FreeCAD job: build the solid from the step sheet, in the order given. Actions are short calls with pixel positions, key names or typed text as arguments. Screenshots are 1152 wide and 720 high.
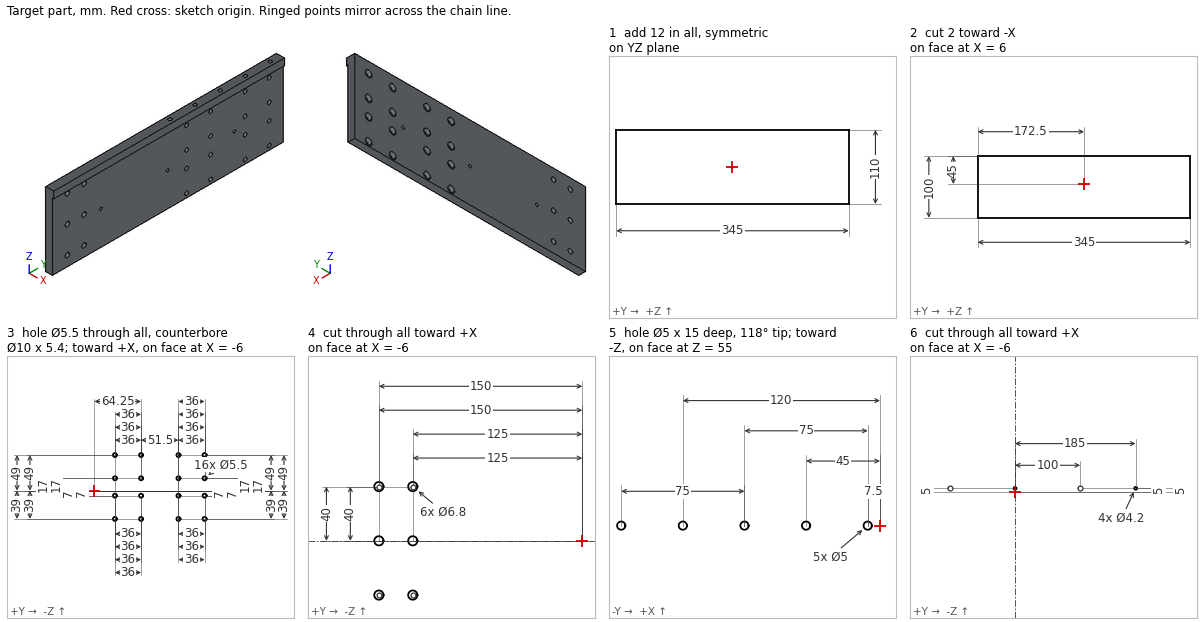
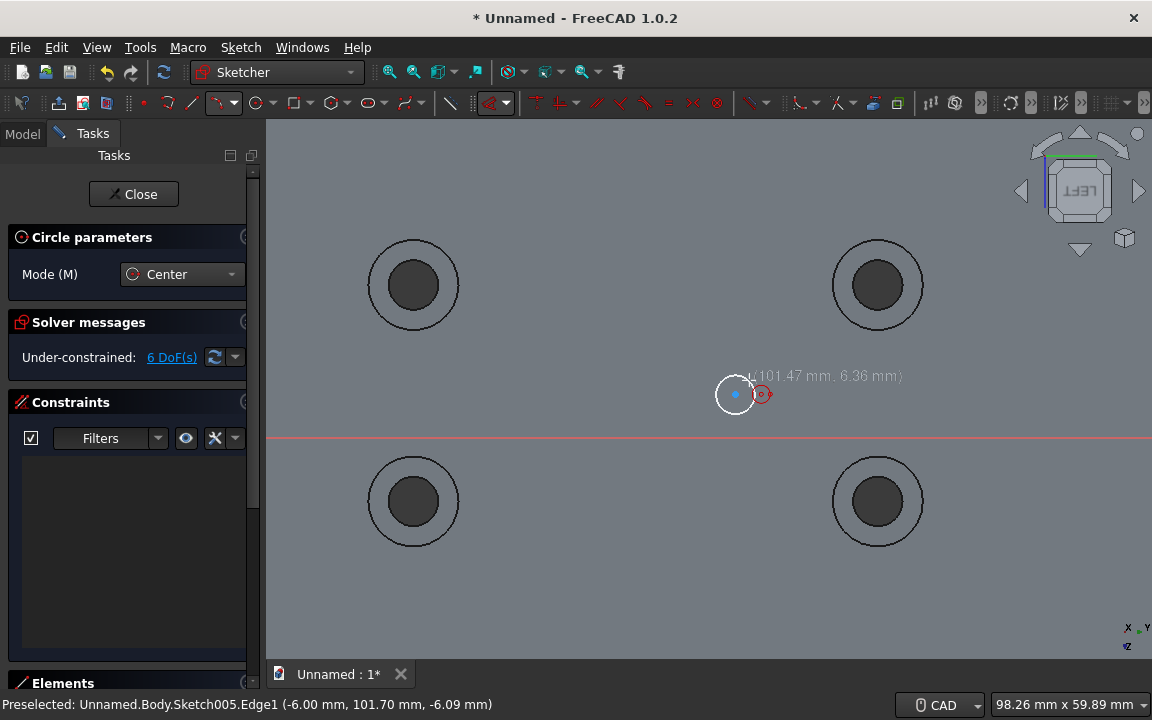
scroll(748, 385, down, 8)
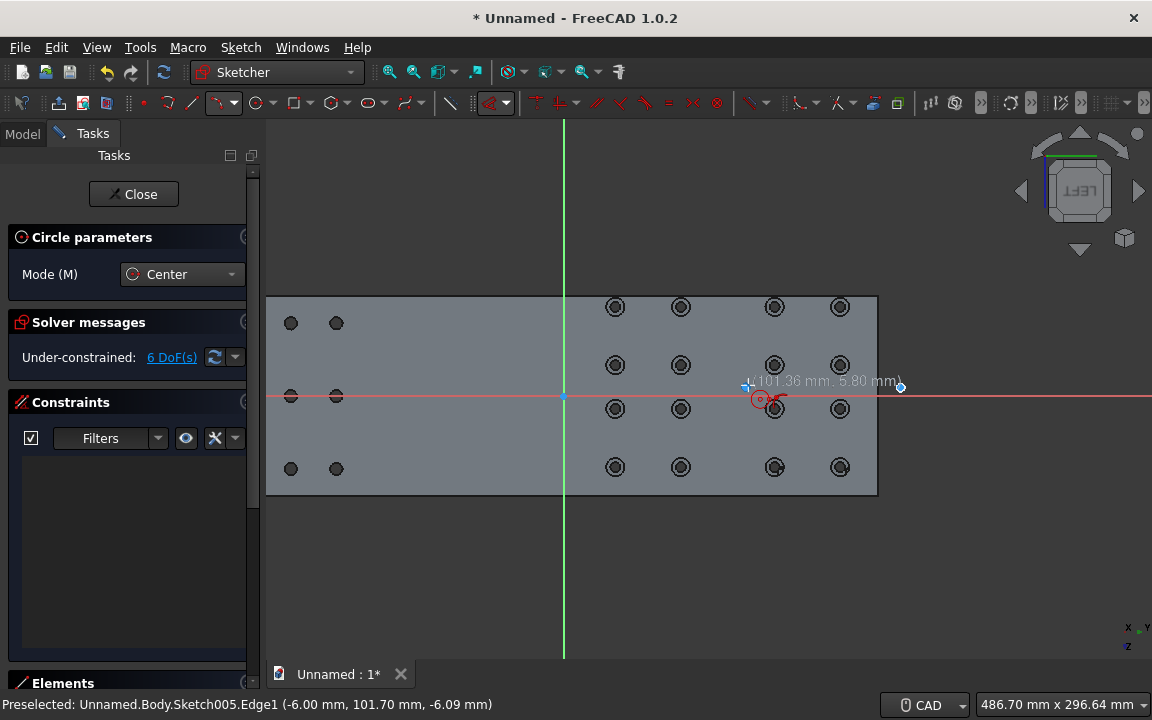
scroll(564, 387, up, 9)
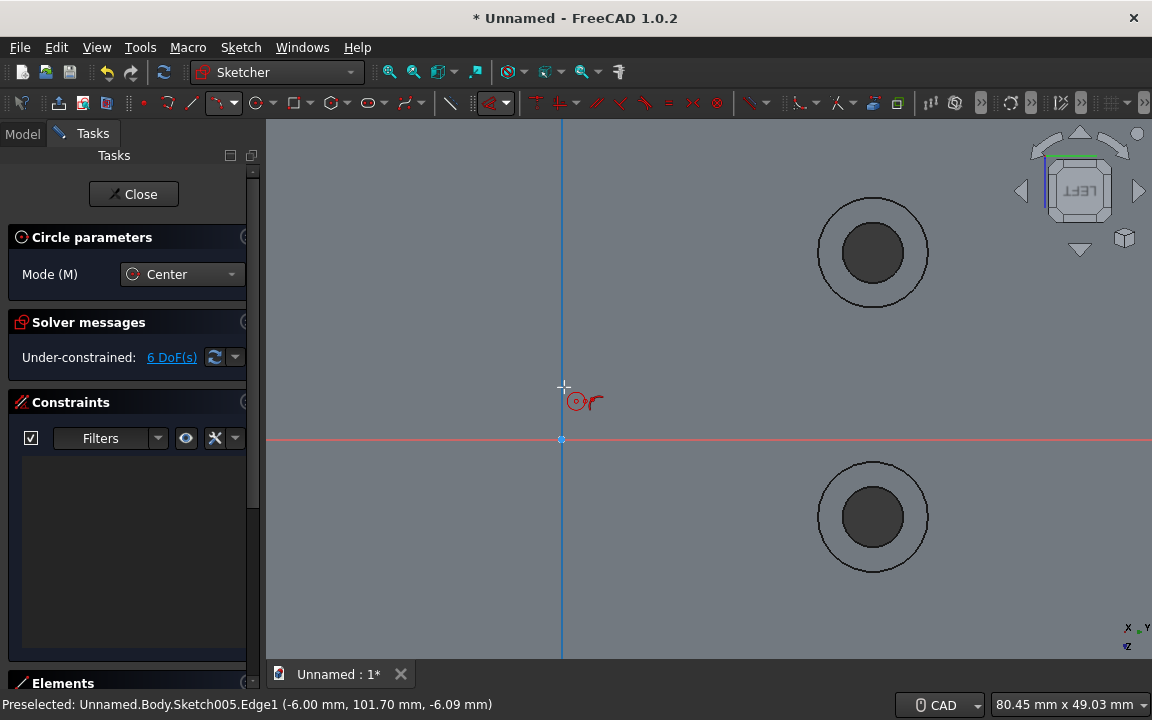
scroll(563, 387, down, 9)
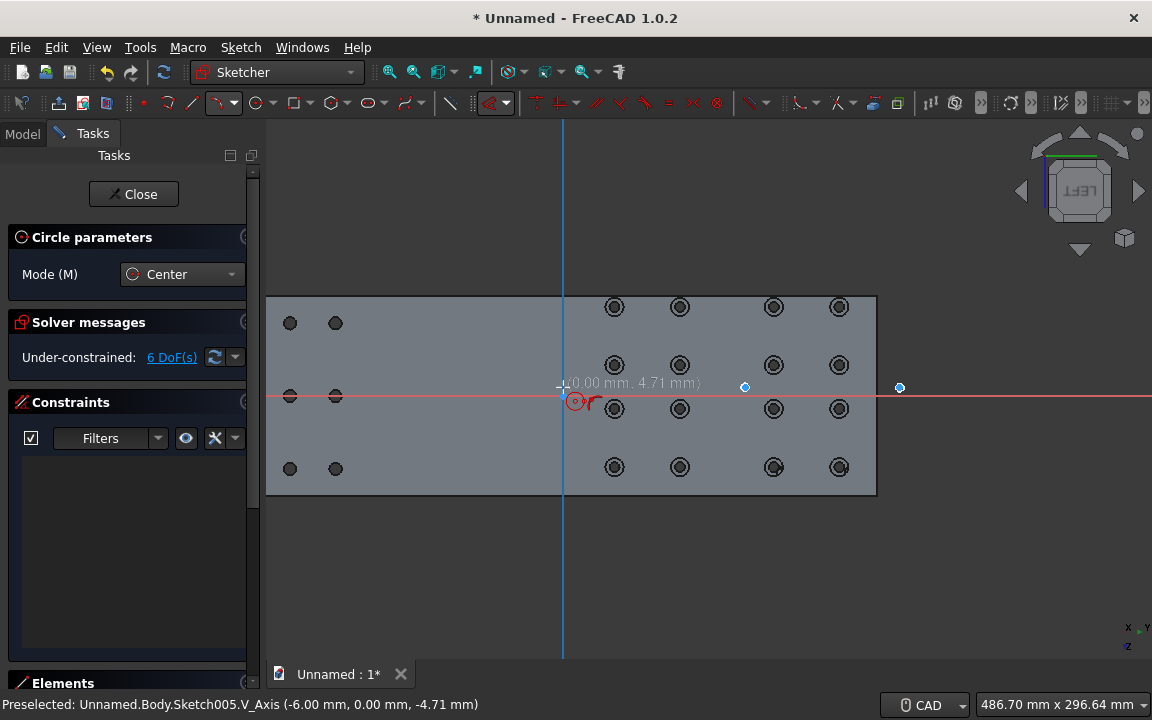
scroll(563, 387, up, 3)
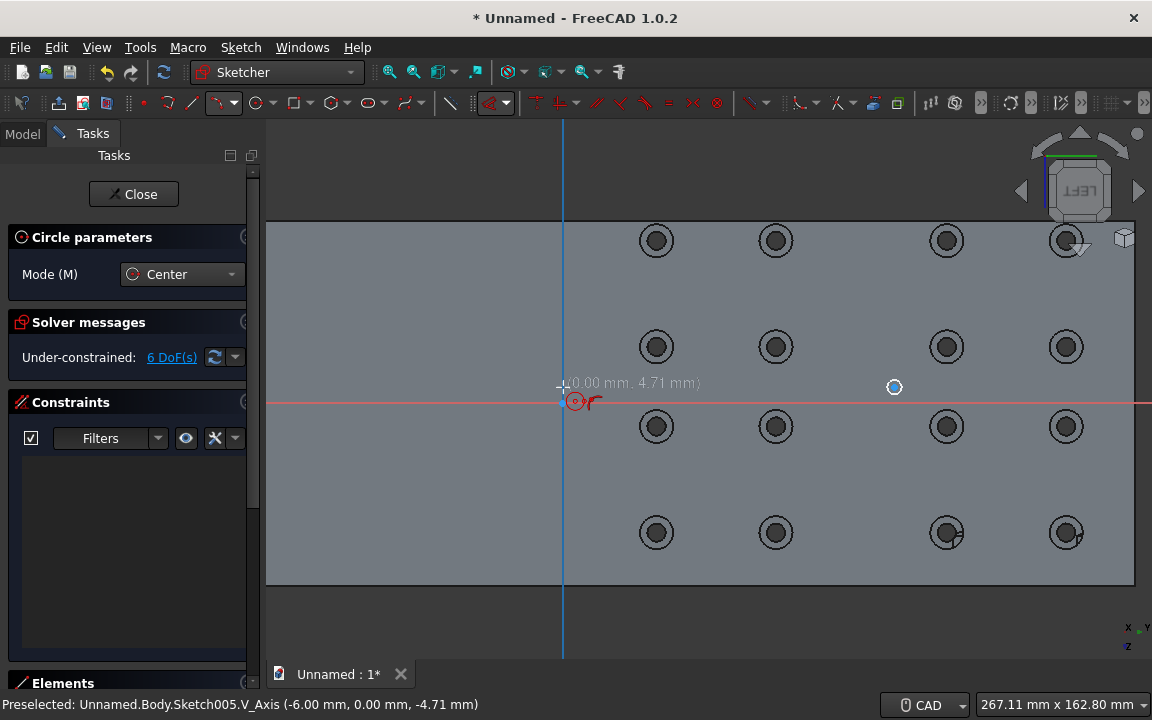
click(563, 387)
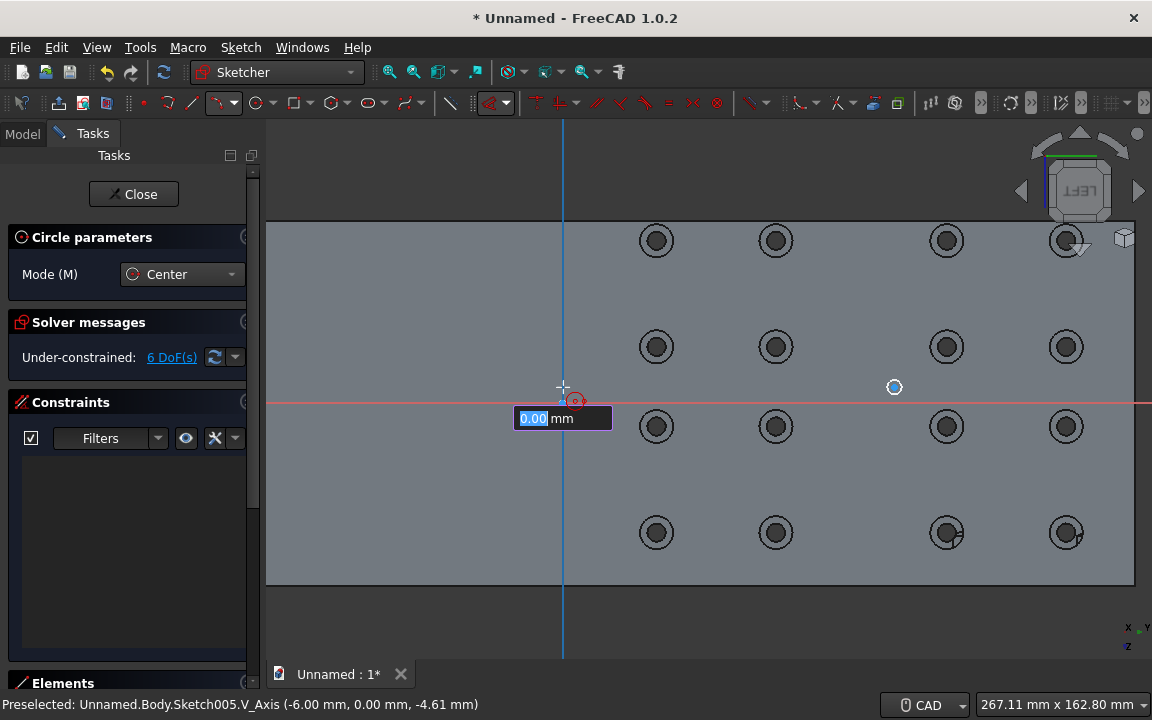
scroll(569, 384, up, 5)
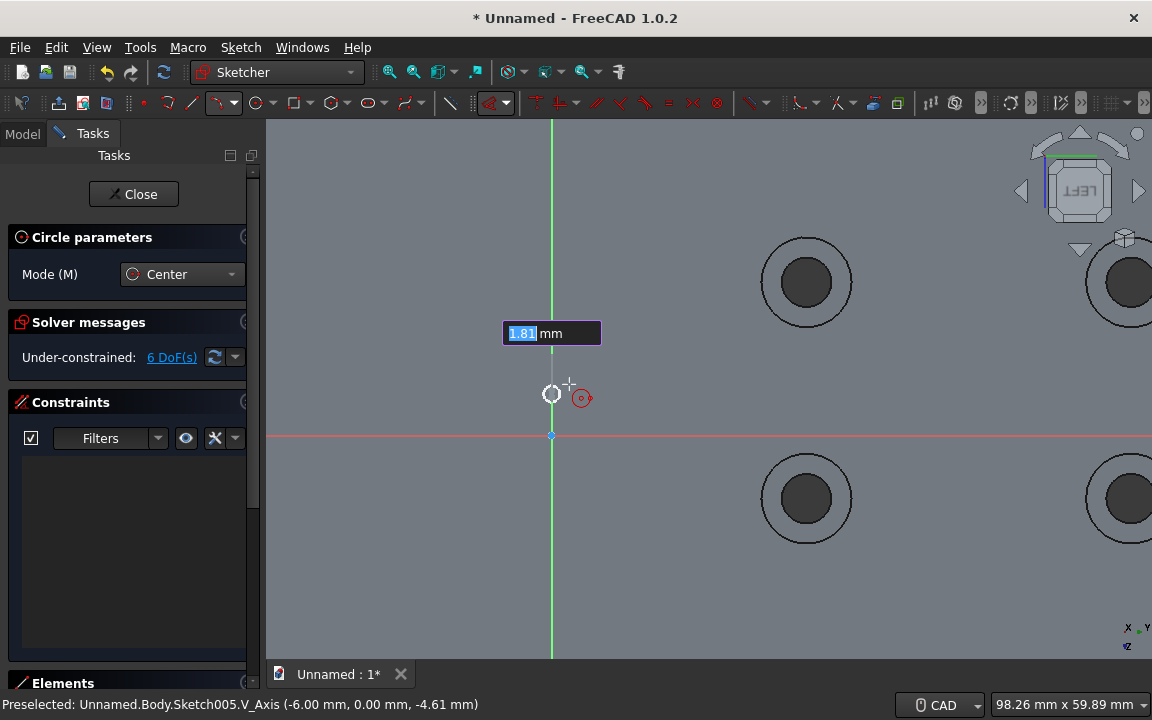
click(570, 384)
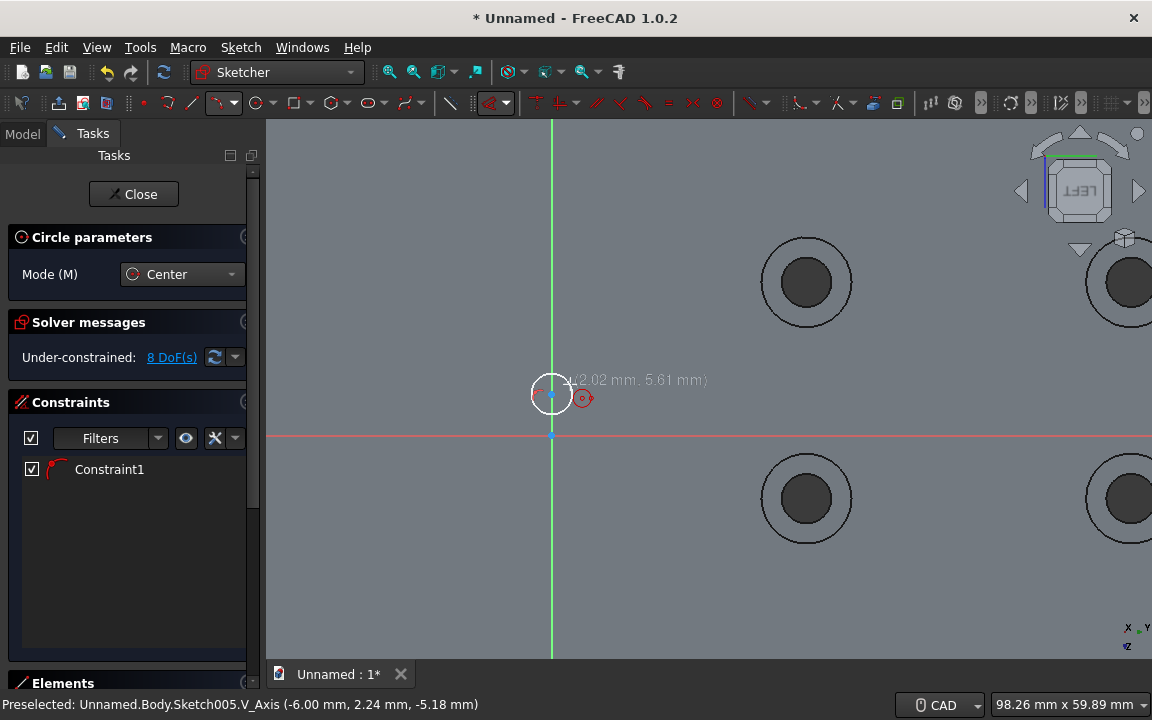
scroll(566, 385, down, 8)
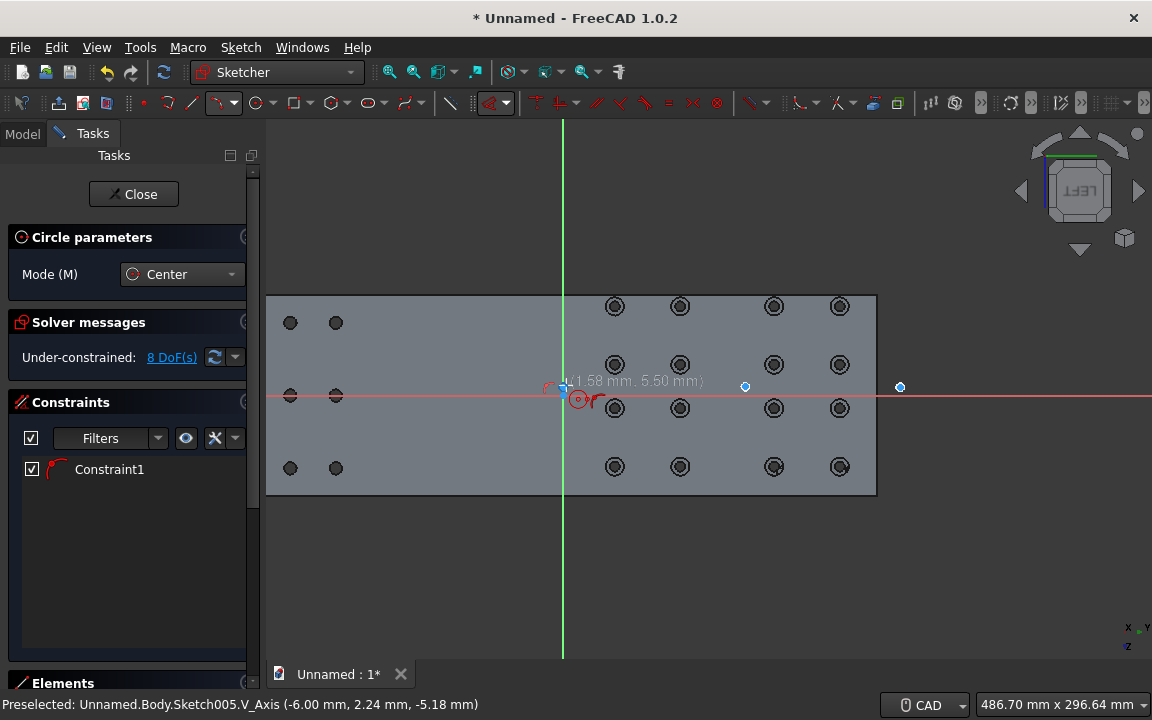
scroll(381, 386, up, 9)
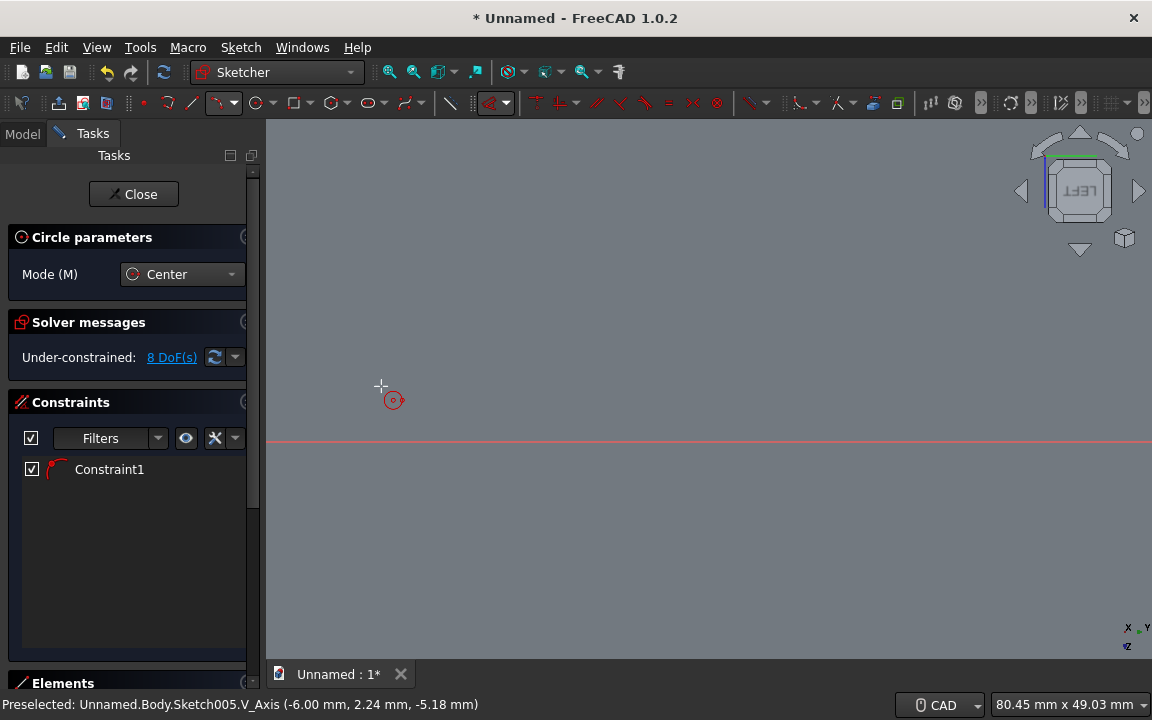
scroll(381, 386, down, 9)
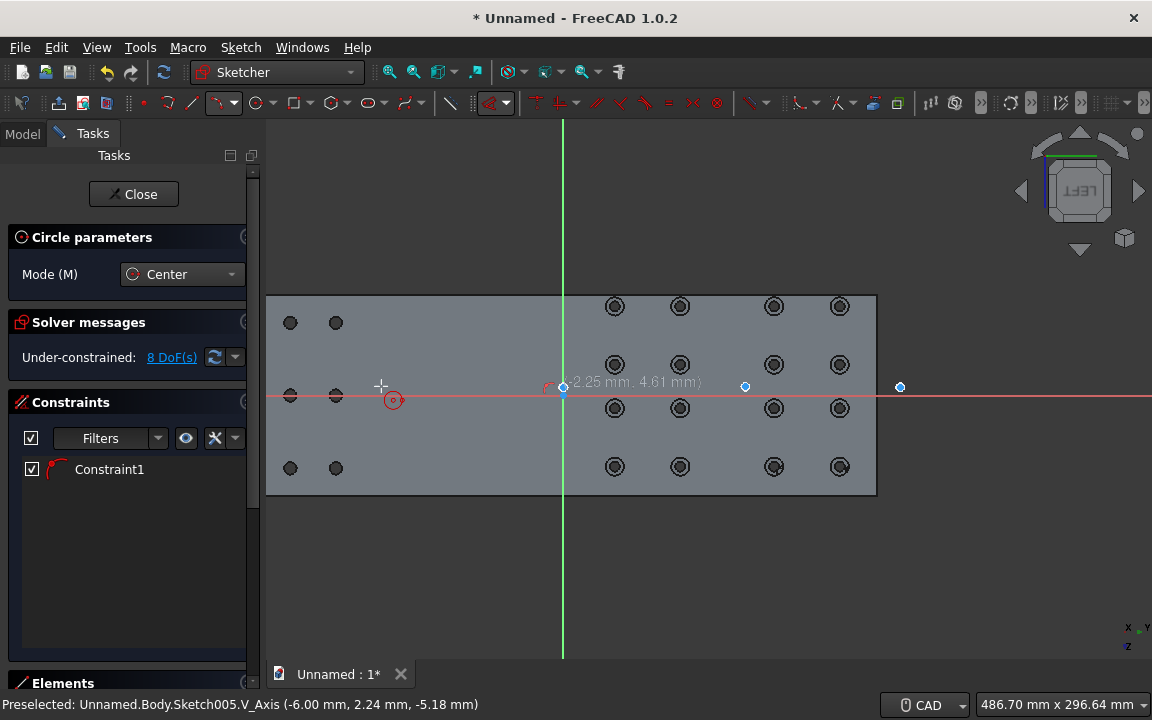
scroll(381, 386, up, 3)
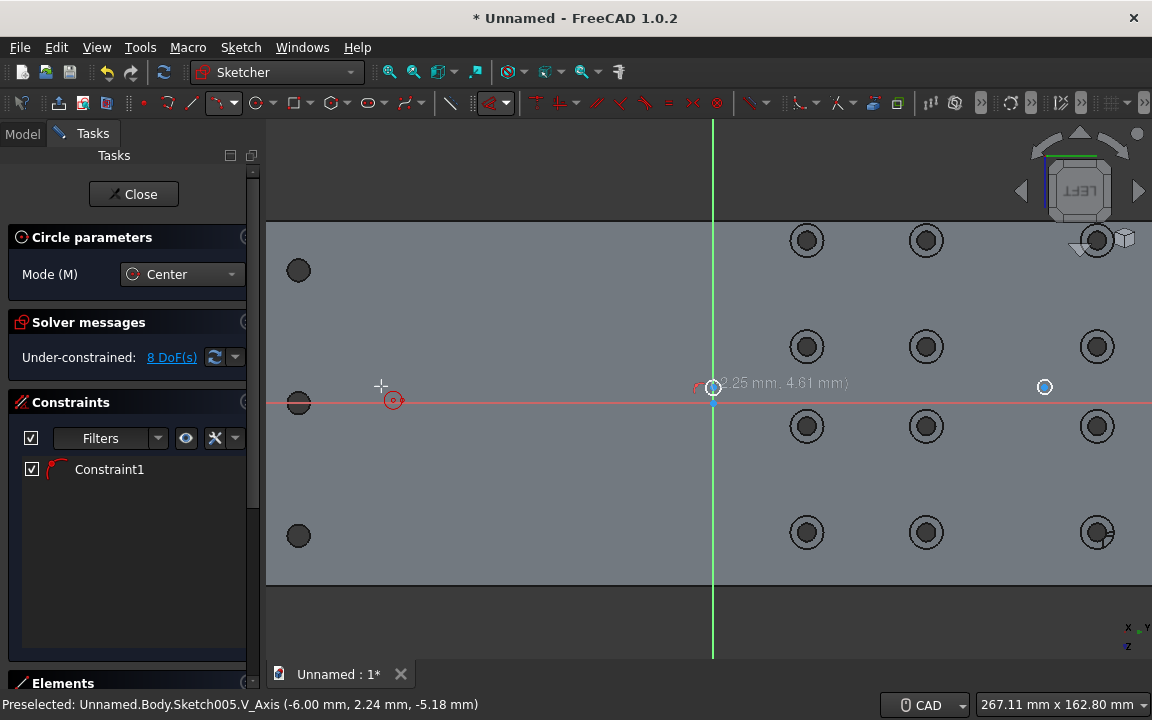
click(382, 387)